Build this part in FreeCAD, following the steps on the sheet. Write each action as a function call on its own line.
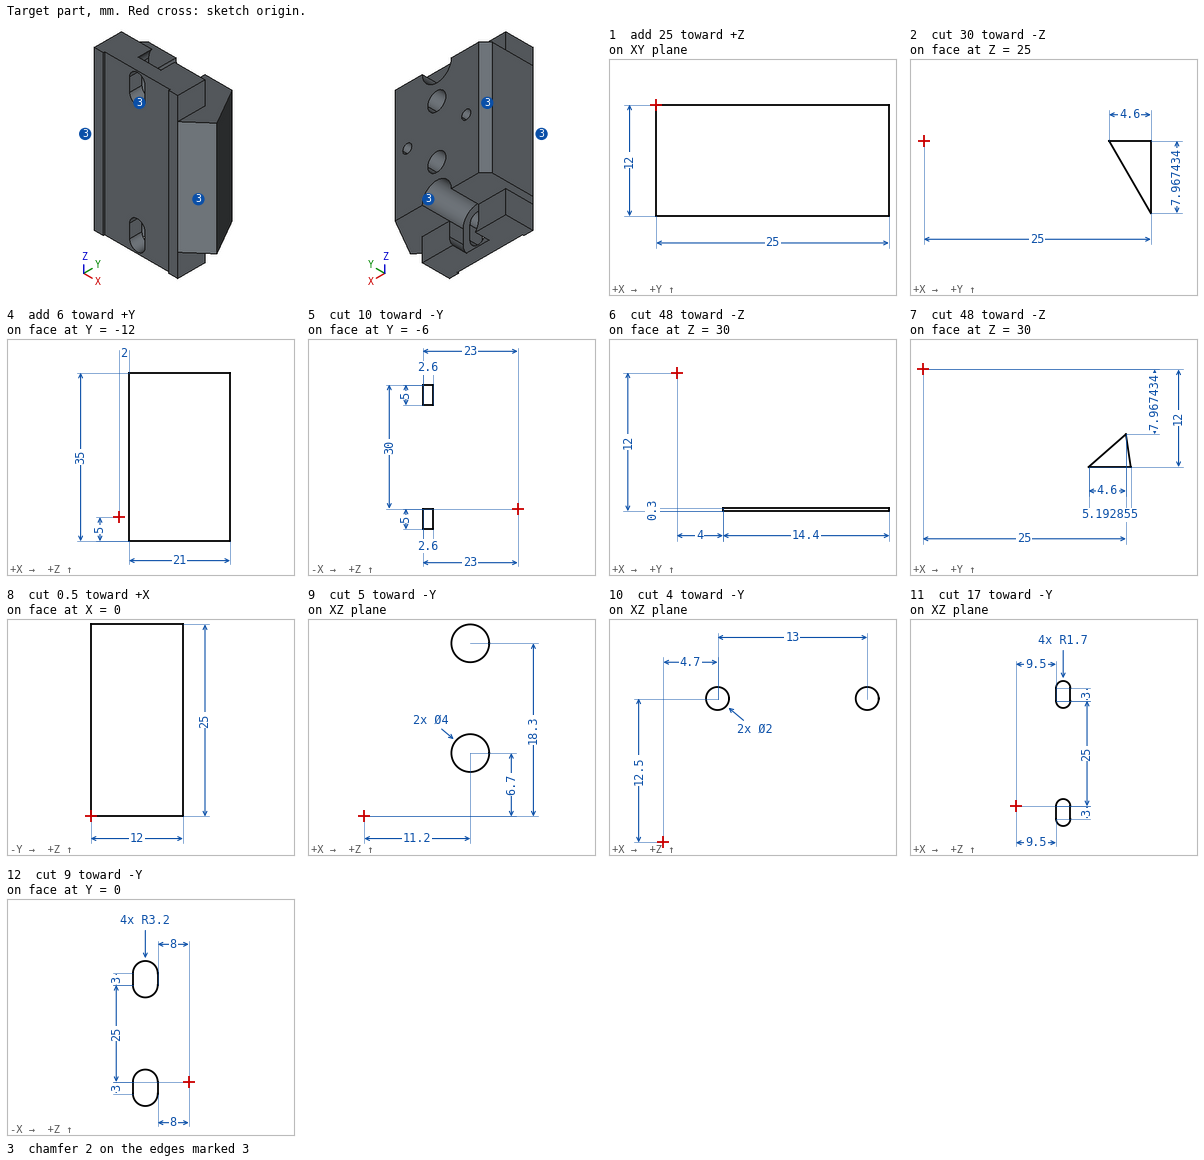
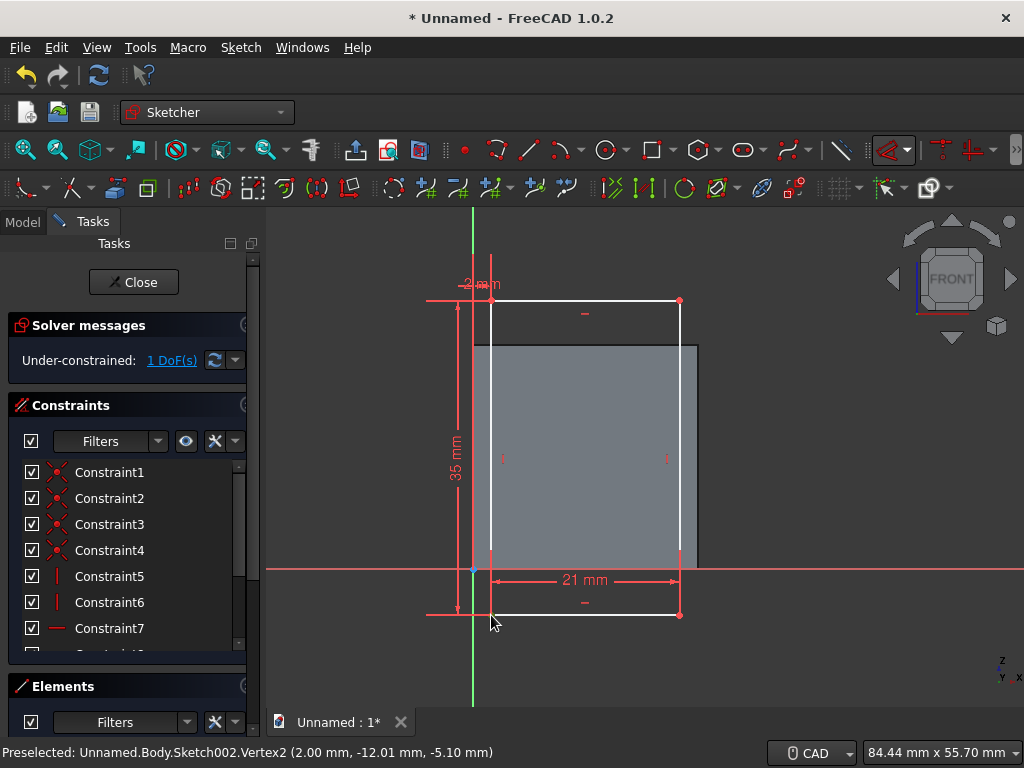
click(910, 150)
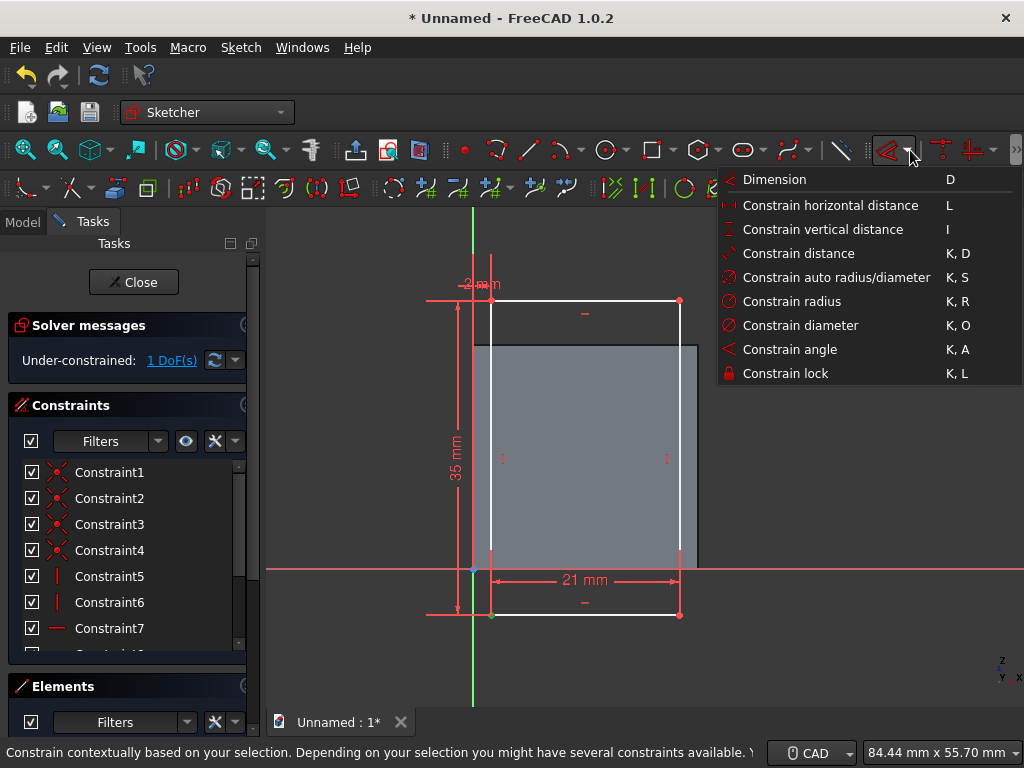
click(870, 229)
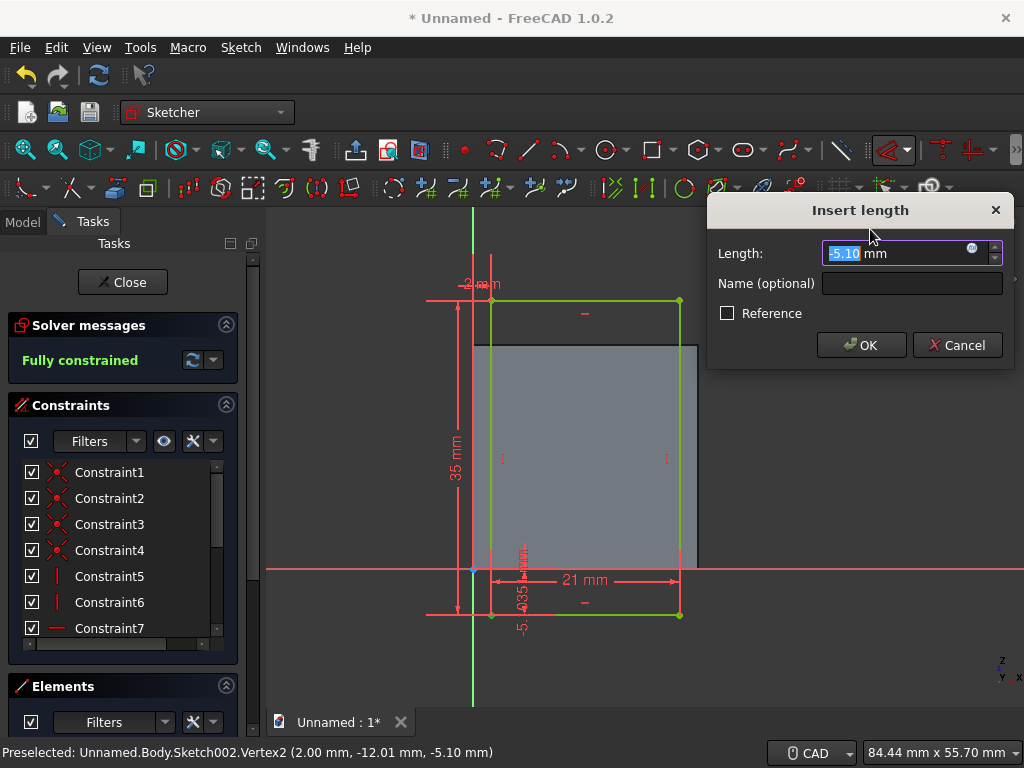
text(-5)
key(Return)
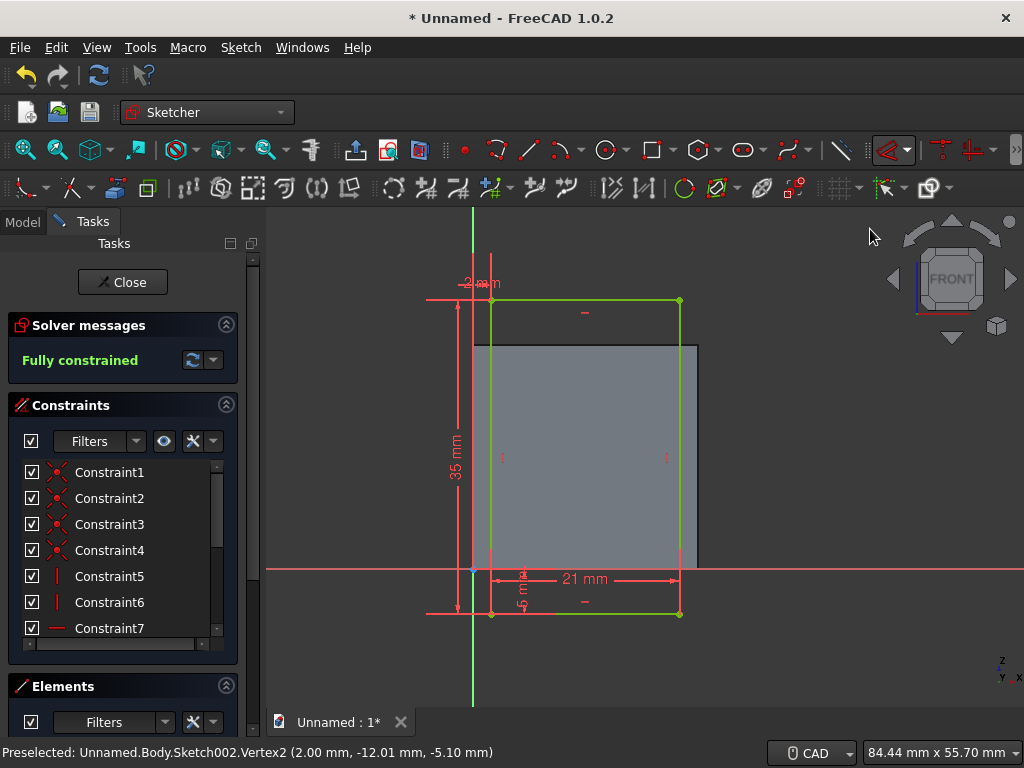
click(123, 282)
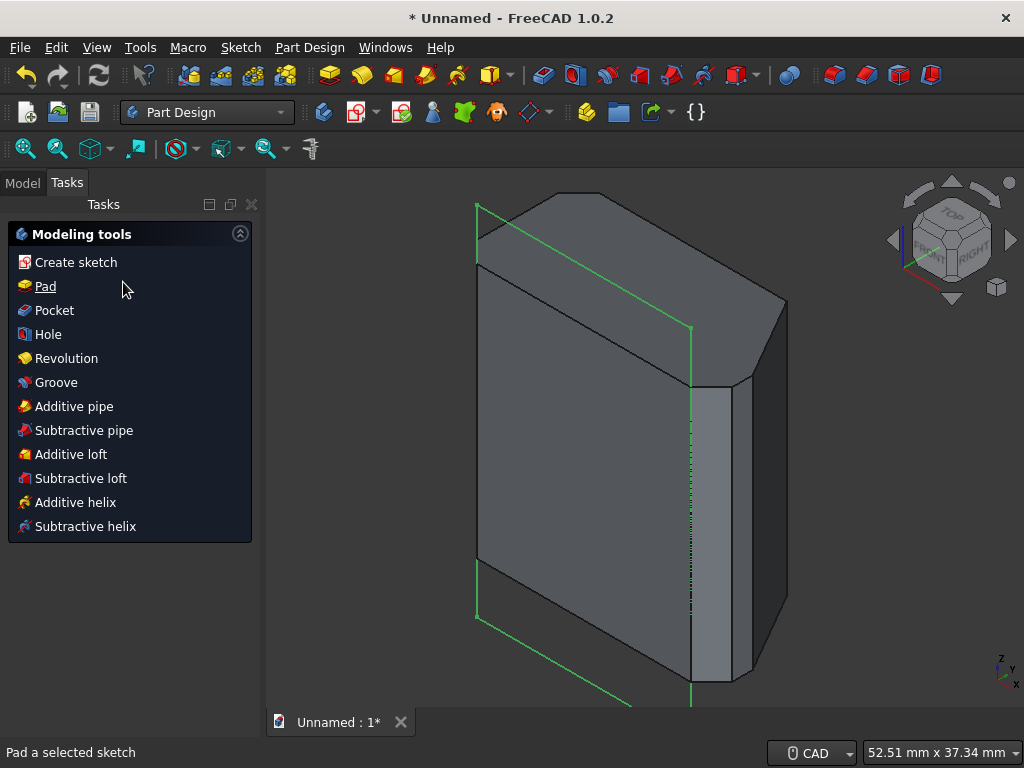
click(330, 76)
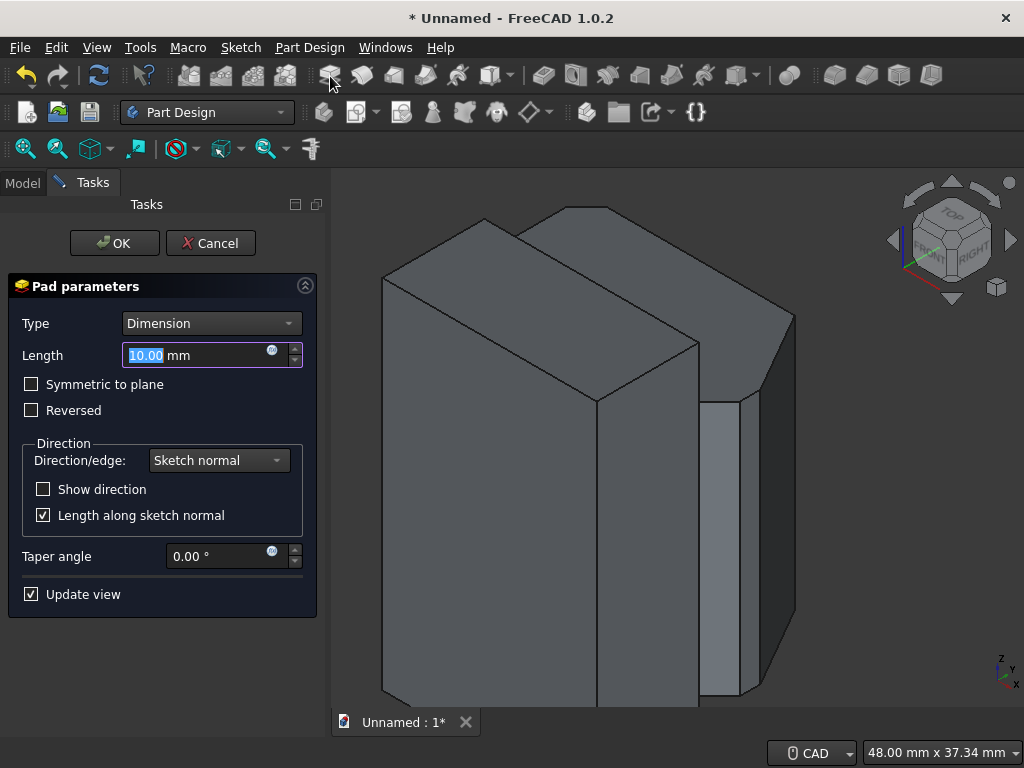
text(6)
key(Tab)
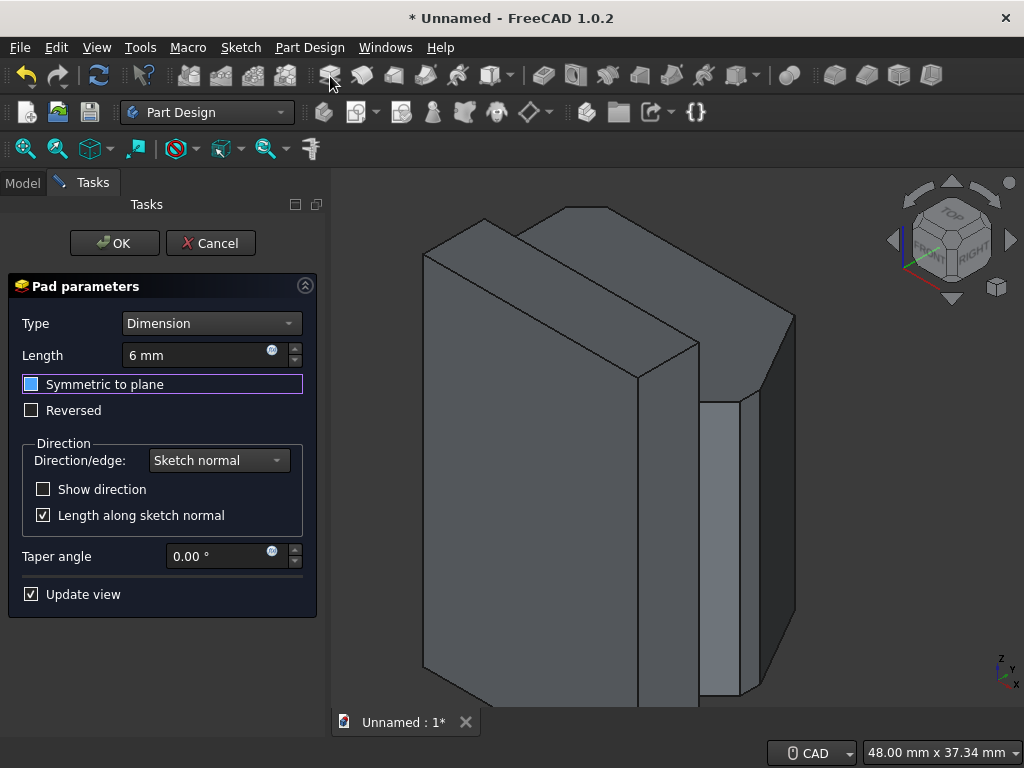
click(30, 410)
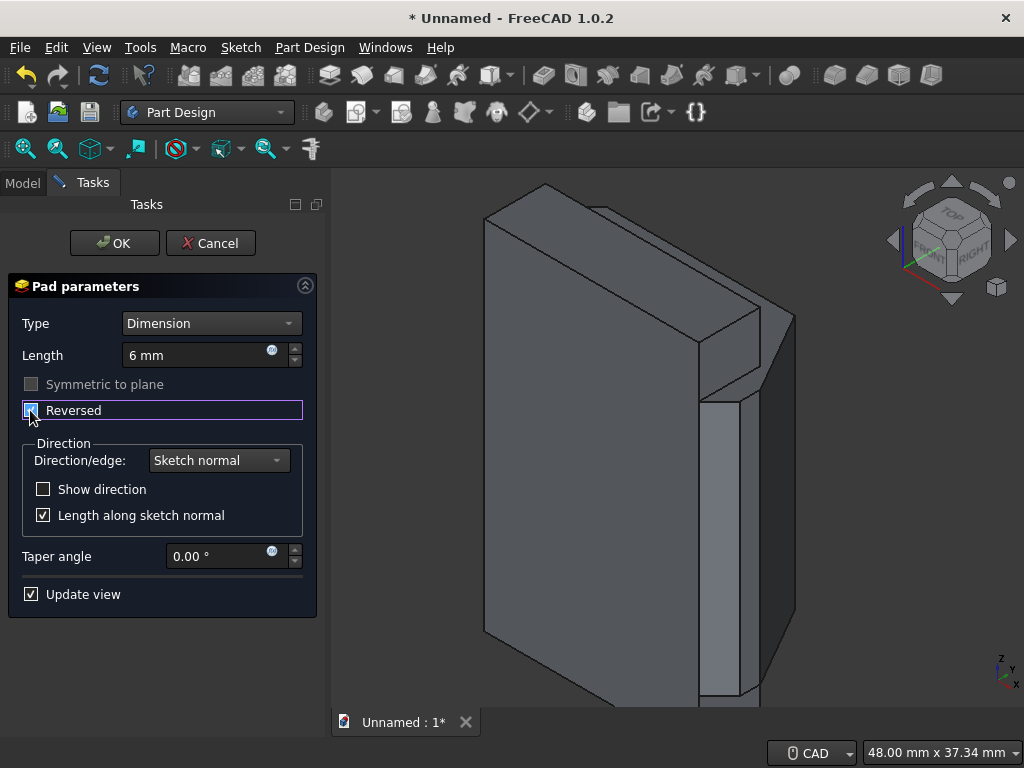
click(115, 243)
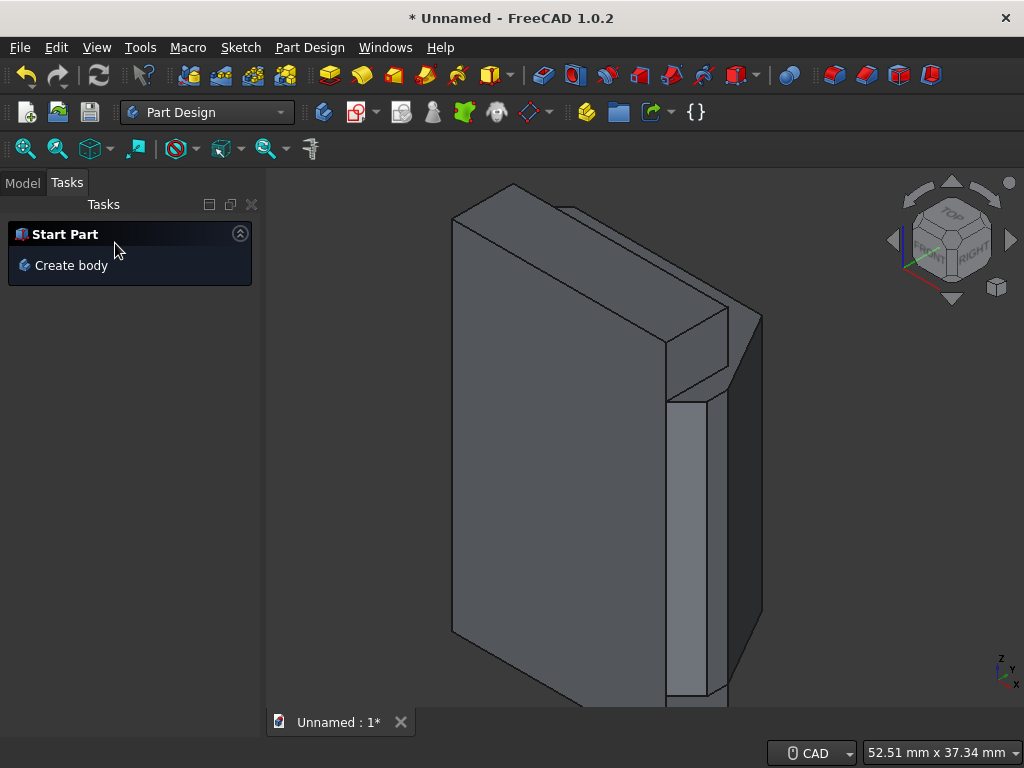
click(26, 150)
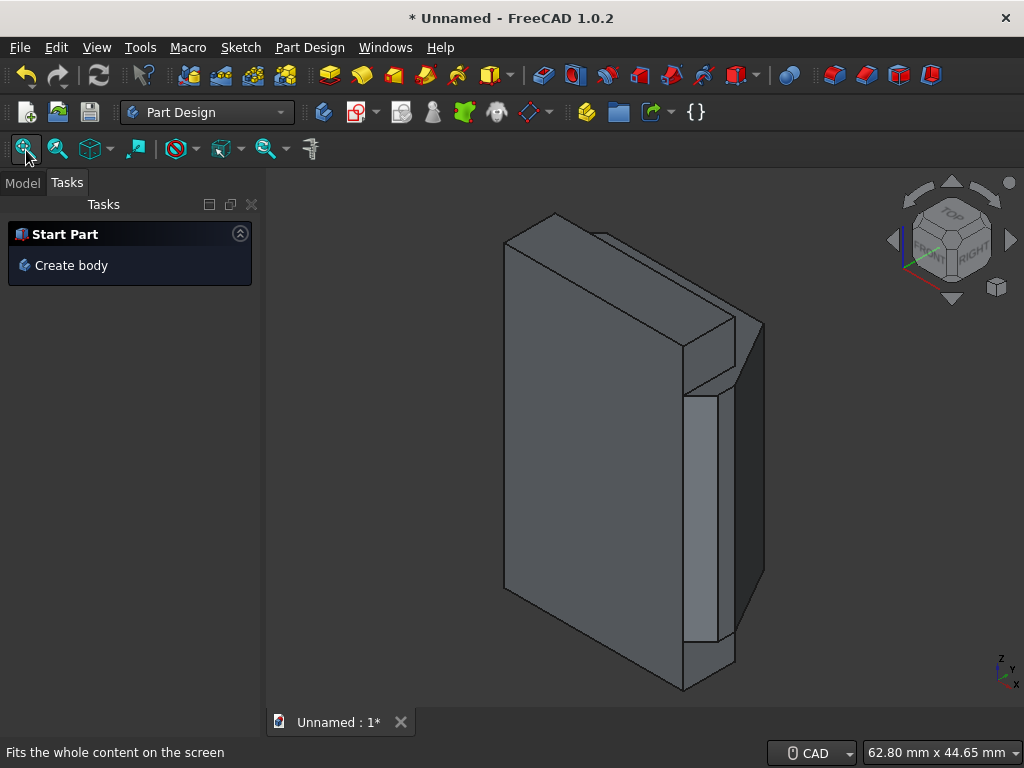
key(4)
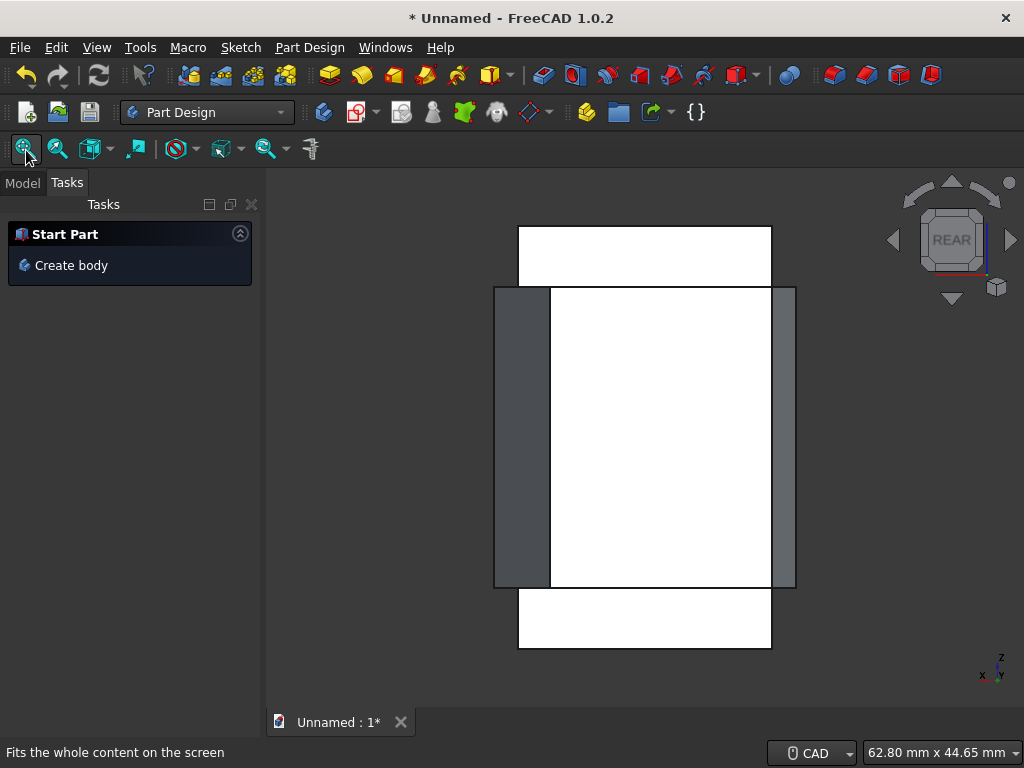
click(573, 618)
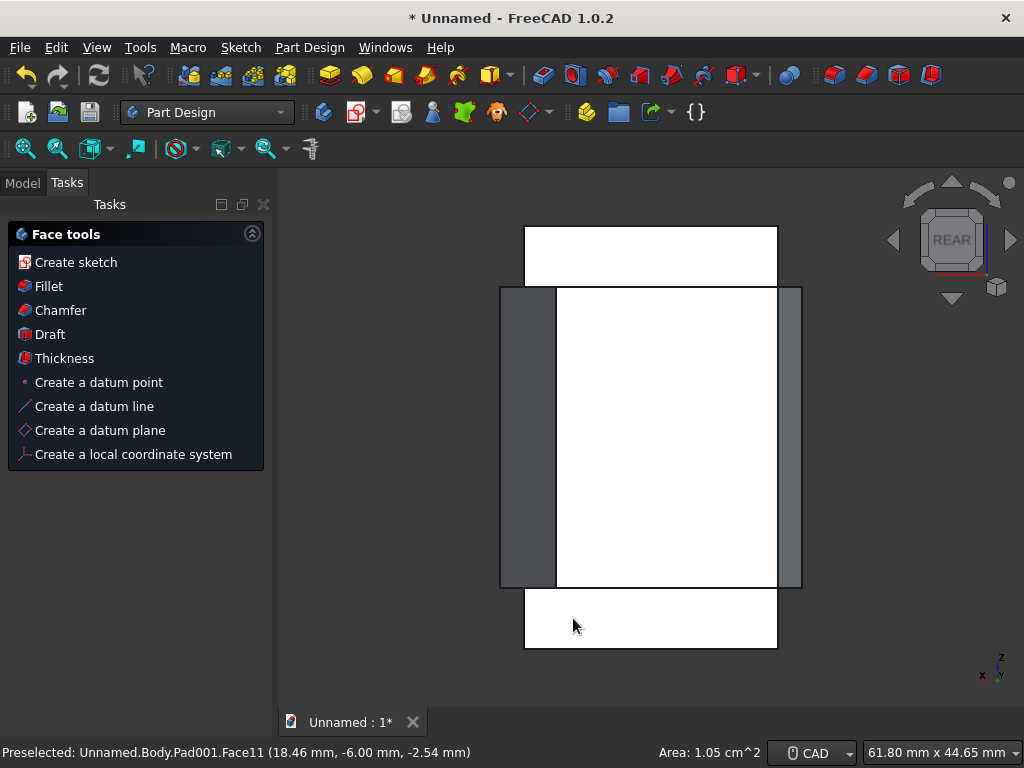
click(356, 112)